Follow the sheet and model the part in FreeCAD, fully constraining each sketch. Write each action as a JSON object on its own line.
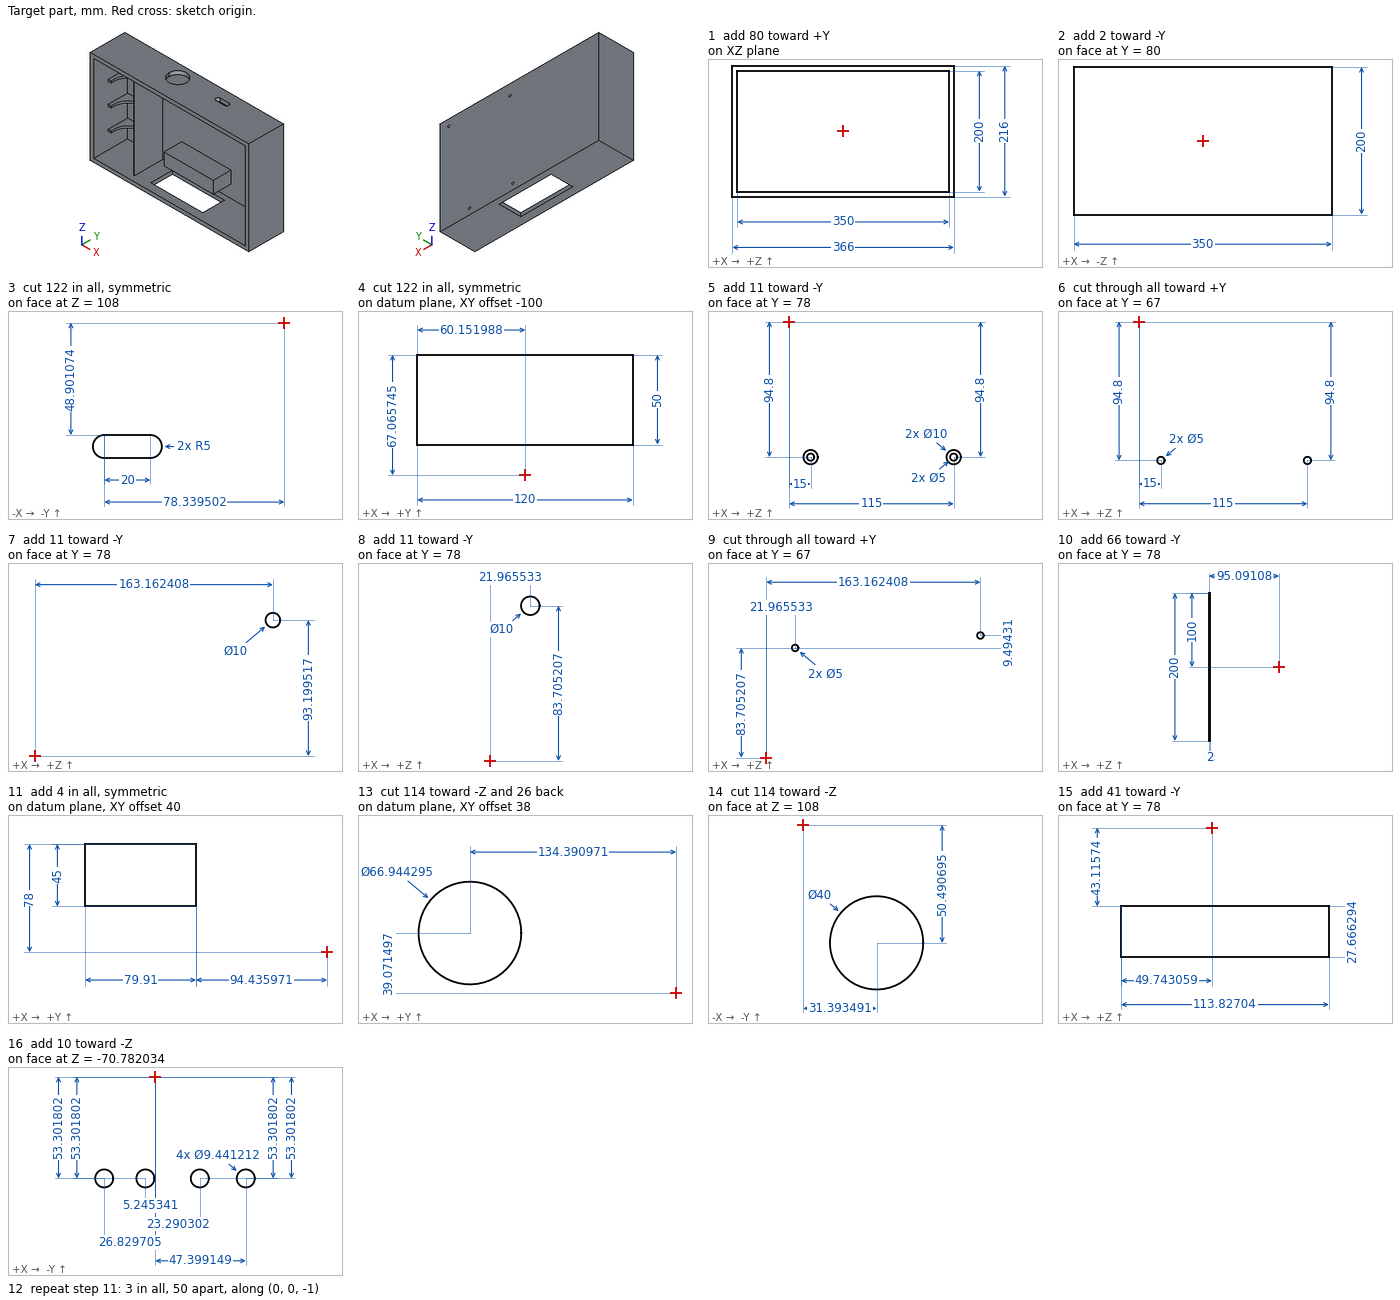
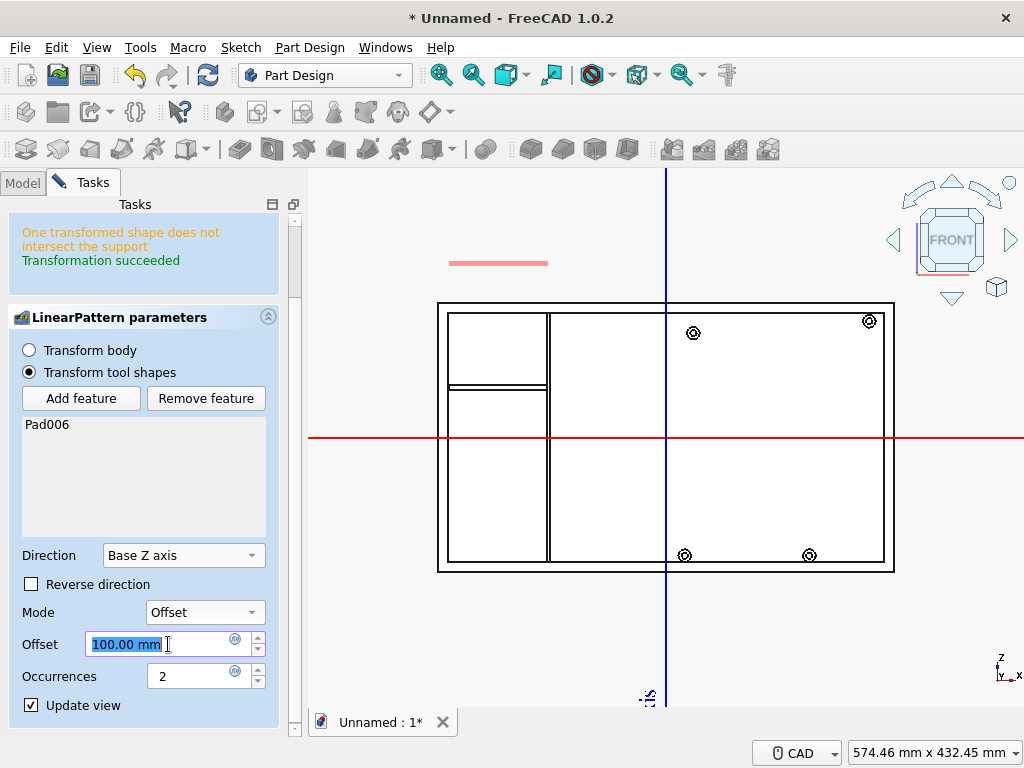
{"action": "type", "text": "50"}
{"action": "key", "text": "Tab"}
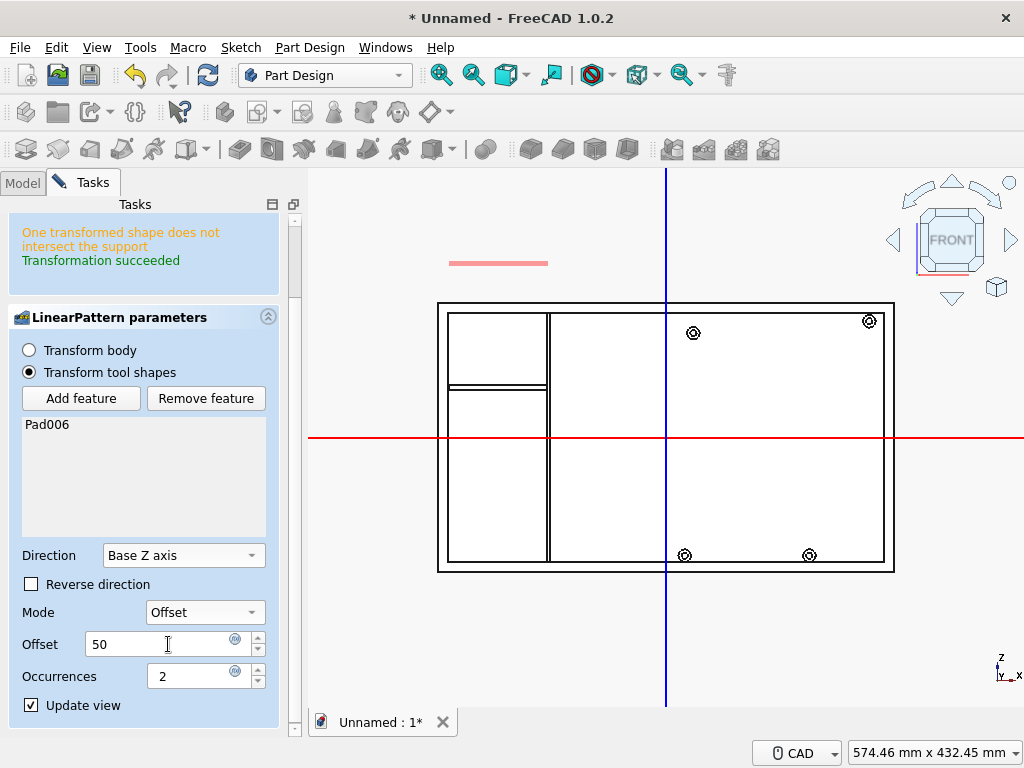
{"action": "triple_click", "coordinate": [198, 676]}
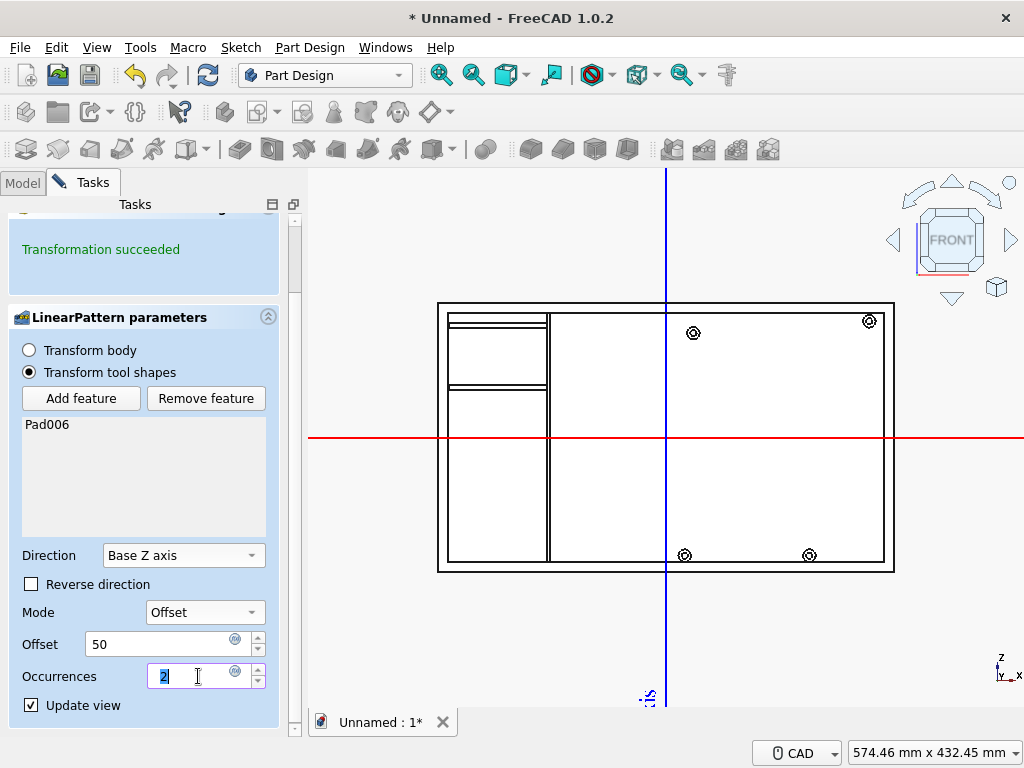
{"action": "type", "text": "3"}
{"action": "key", "text": "Tab"}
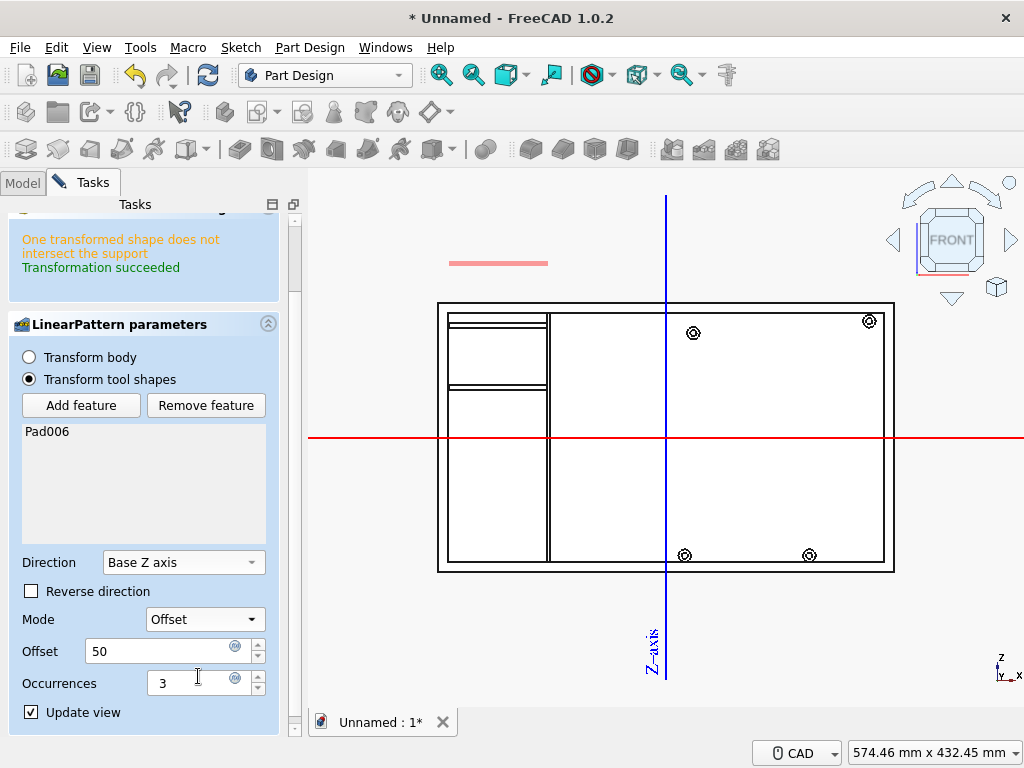
{"action": "left_click", "coordinate": [30, 591]}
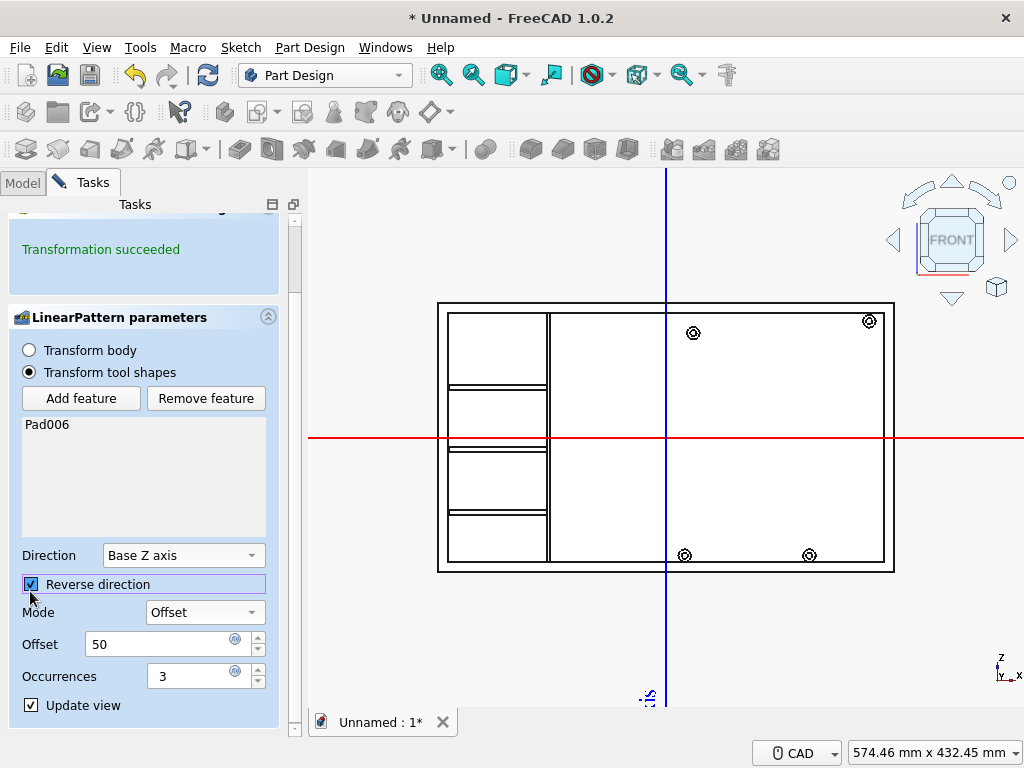
{"action": "scroll", "coordinate": [295, 475], "scroll_direction": "up", "scroll_amount": 3}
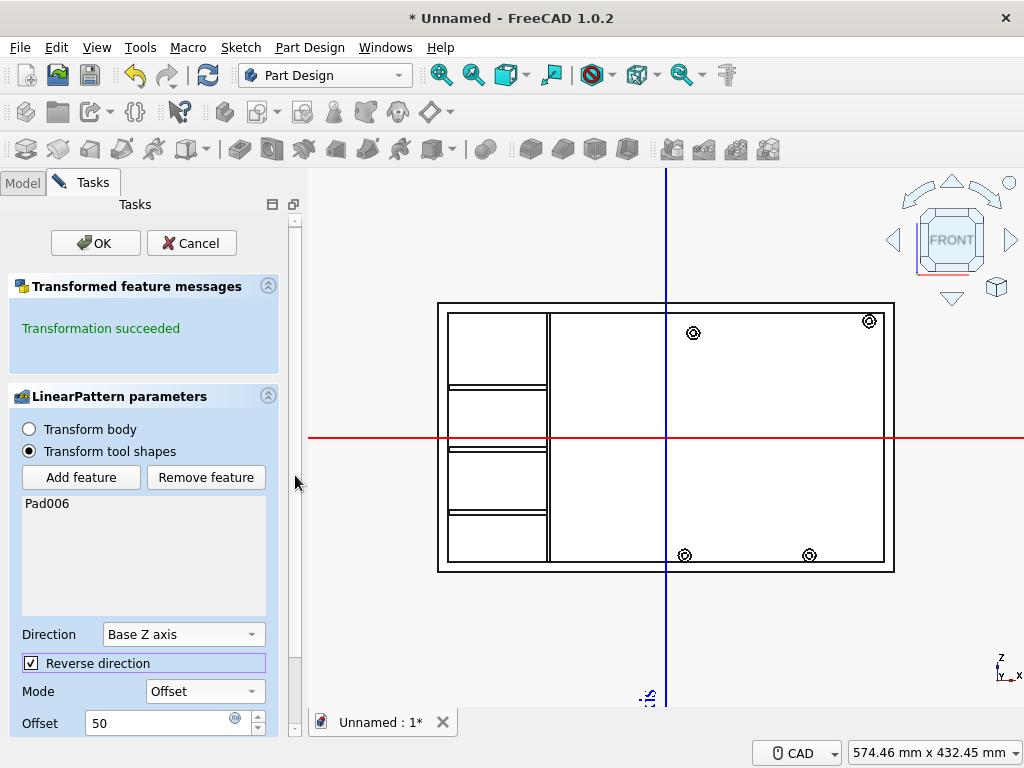
{"action": "left_click", "coordinate": [96, 243]}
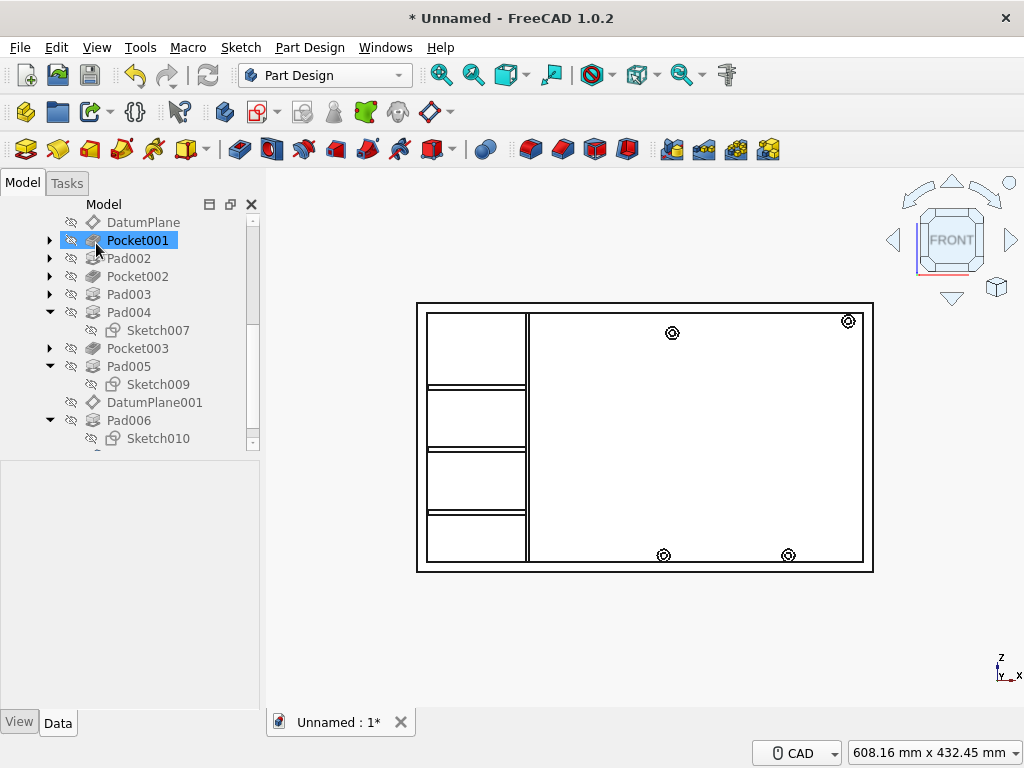
{"action": "scroll", "coordinate": [140, 326], "scroll_direction": "down", "scroll_amount": 3}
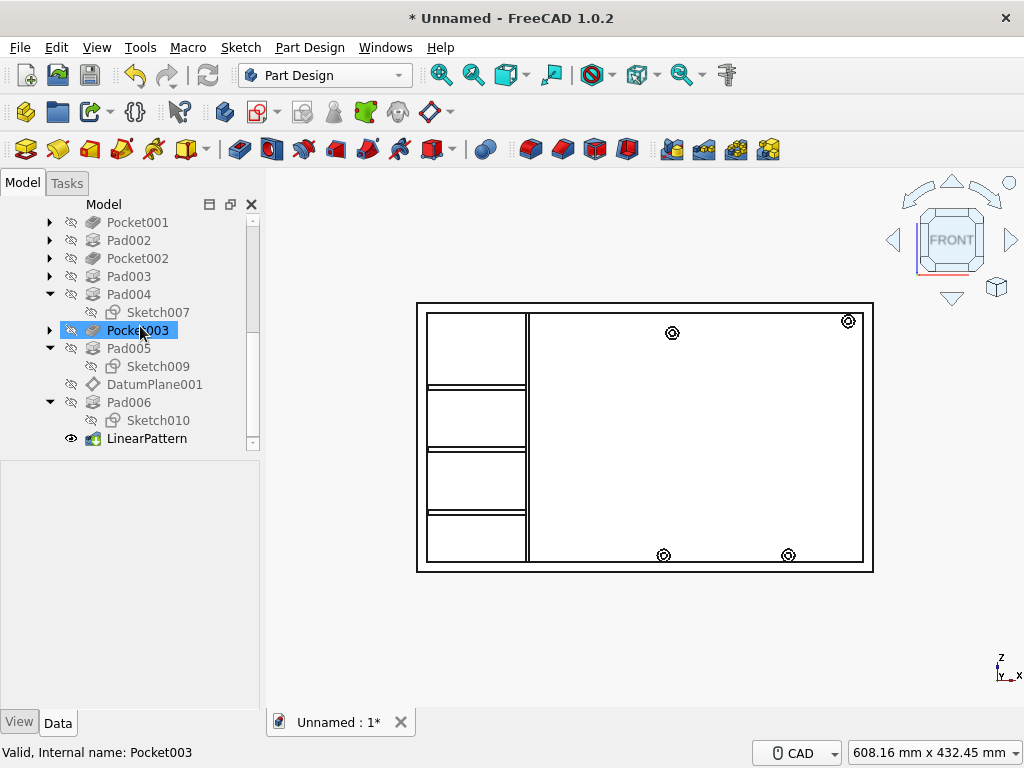
{"action": "scroll", "coordinate": [140, 326], "scroll_direction": "up", "scroll_amount": 15}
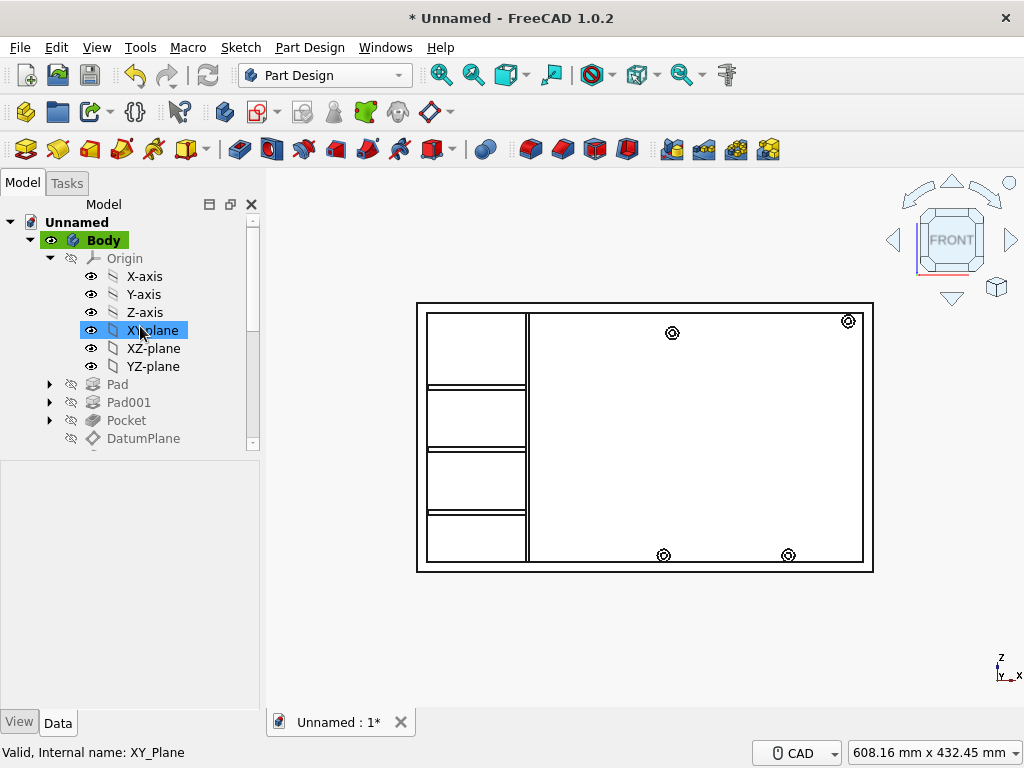
{"action": "left_click", "coordinate": [136, 330]}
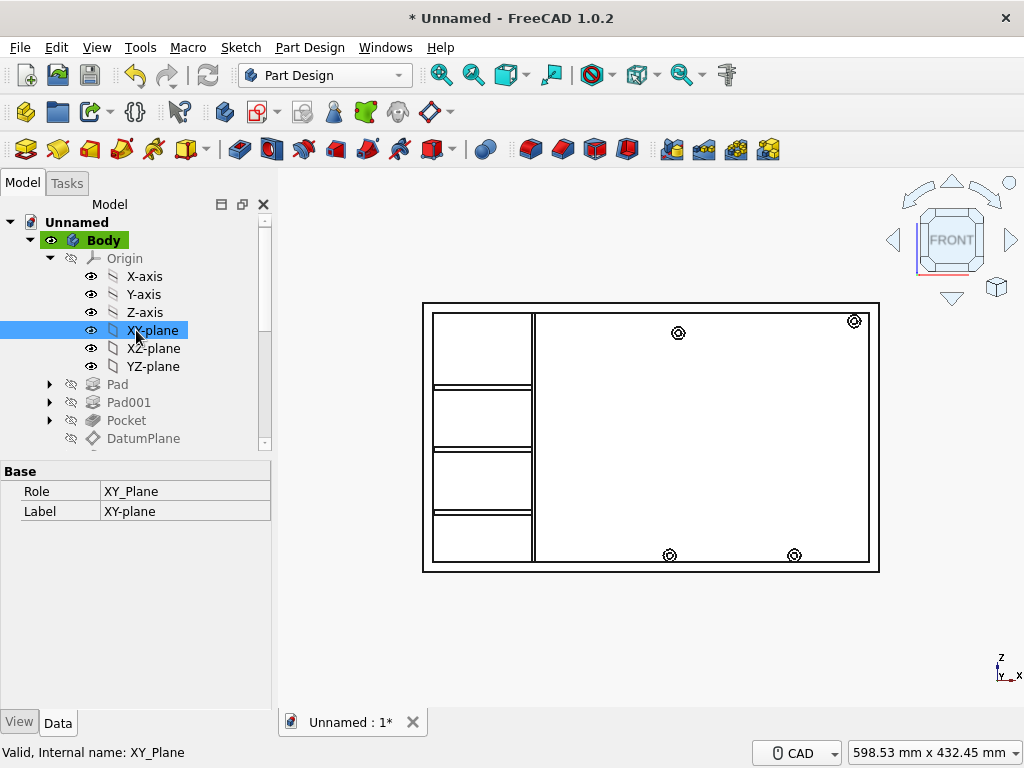
{"action": "left_click", "coordinate": [430, 112]}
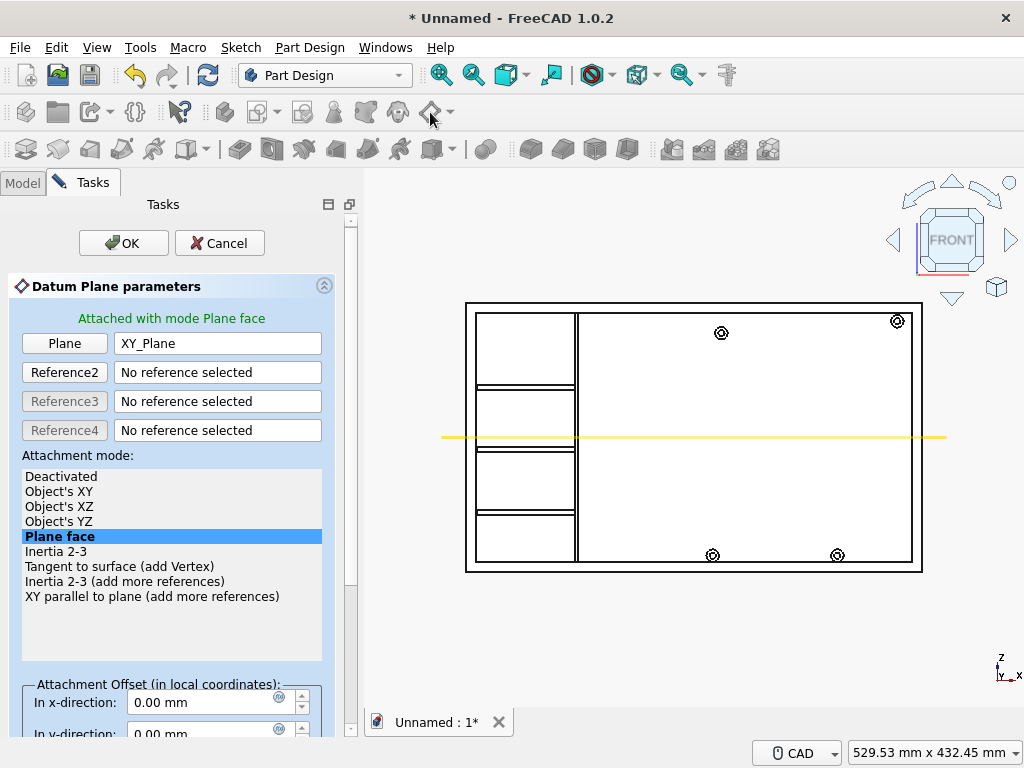
{"action": "scroll", "coordinate": [351, 475], "scroll_direction": "down", "scroll_amount": 2}